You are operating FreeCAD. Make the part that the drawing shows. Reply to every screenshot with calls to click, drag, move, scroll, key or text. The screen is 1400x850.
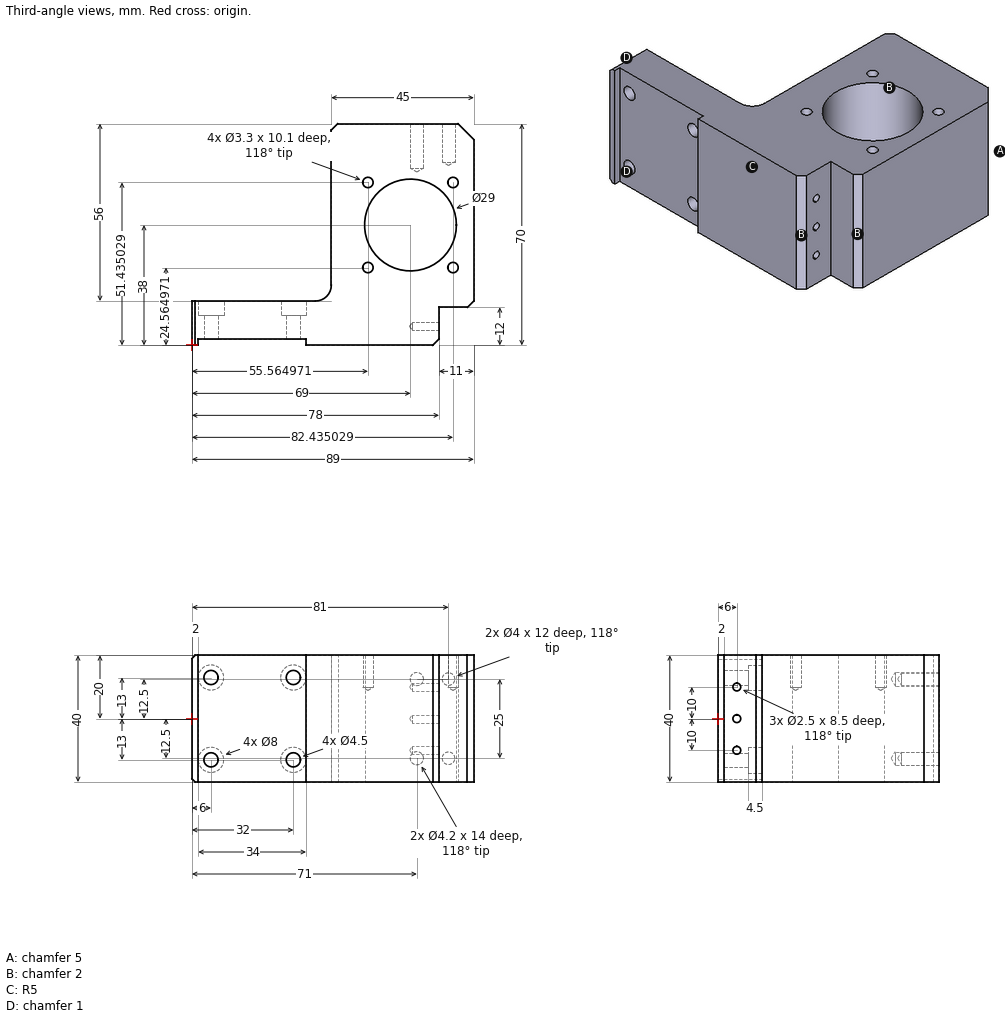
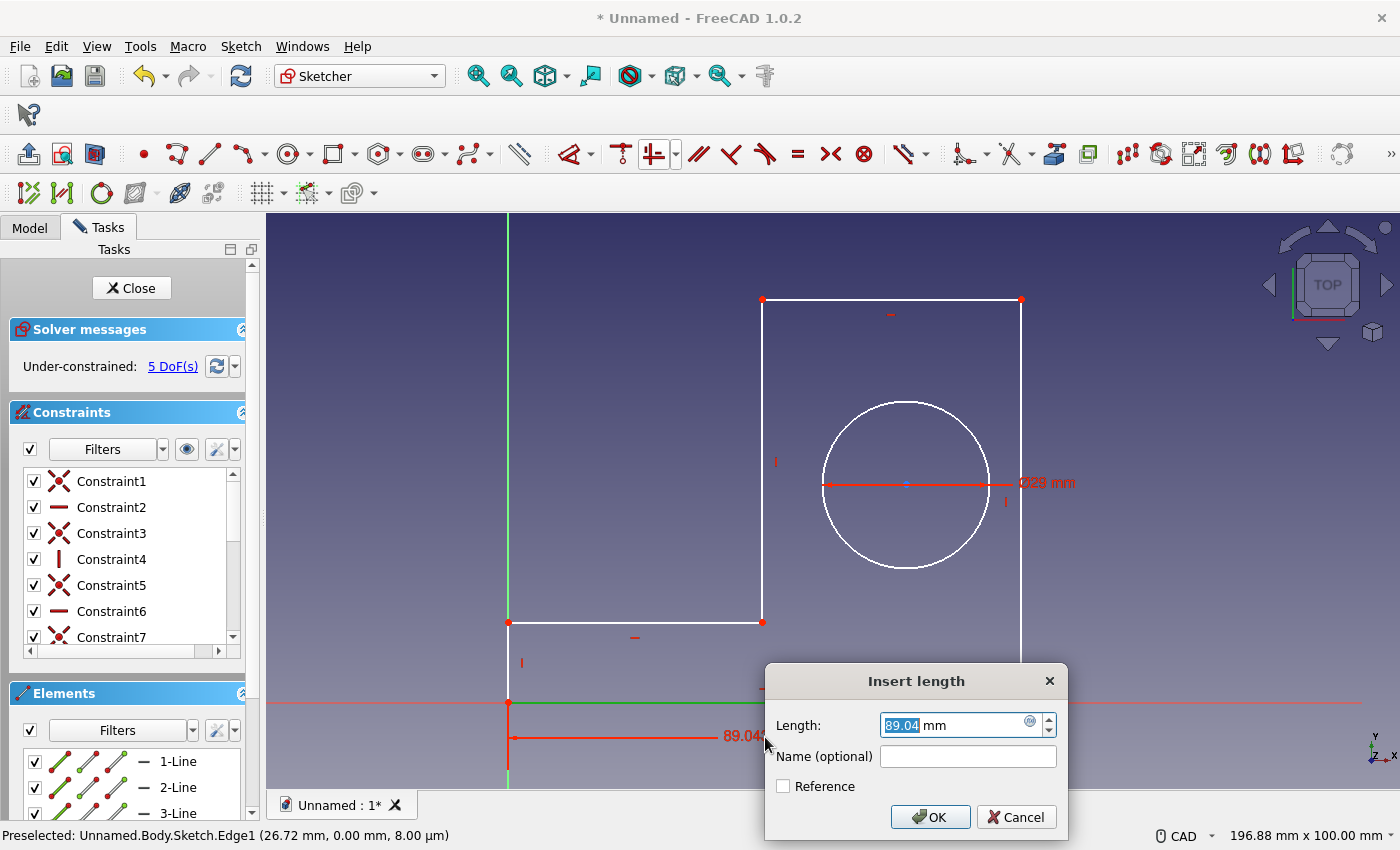
text(89)
key(Return)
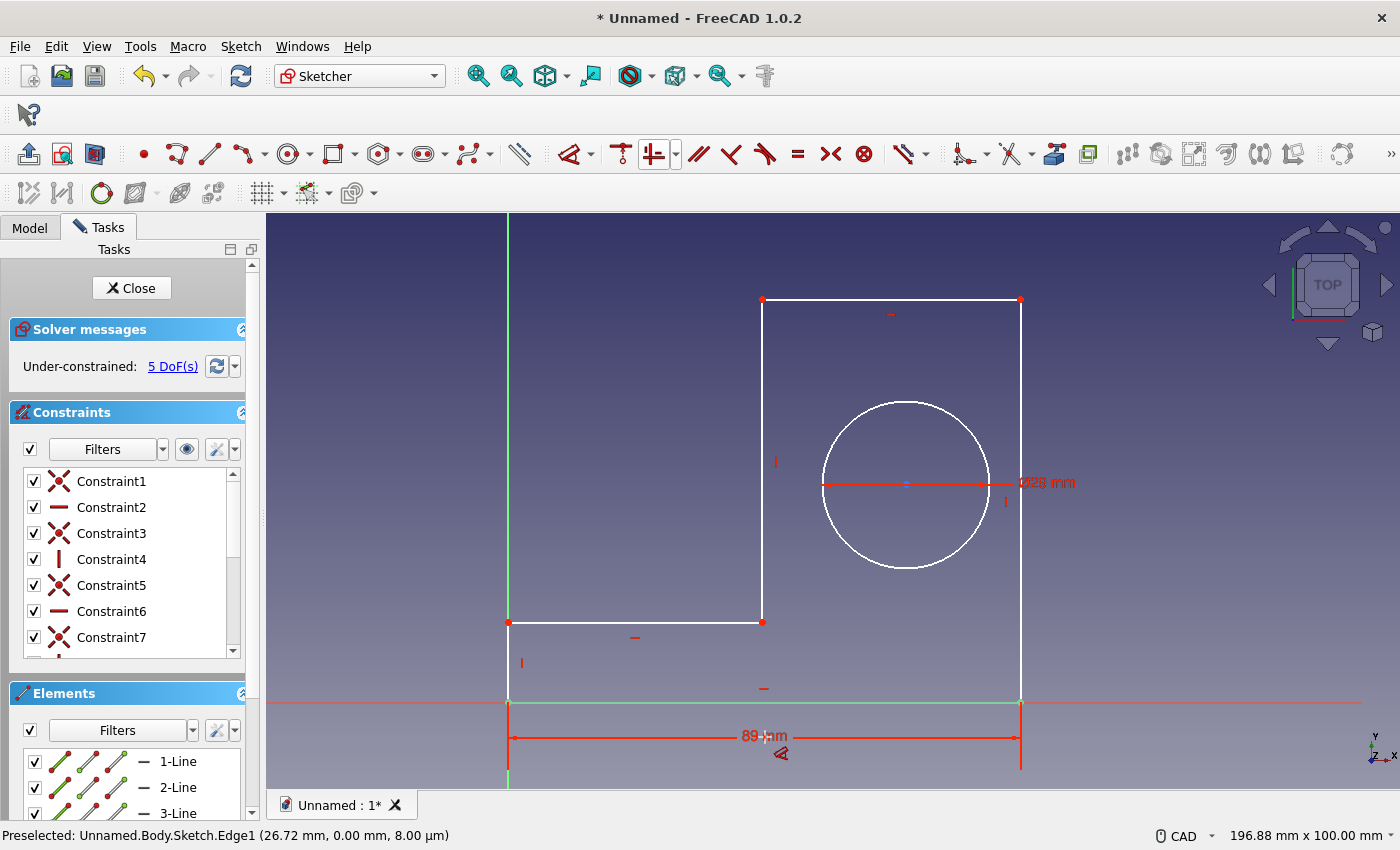
click(1021, 582)
click(1055, 501)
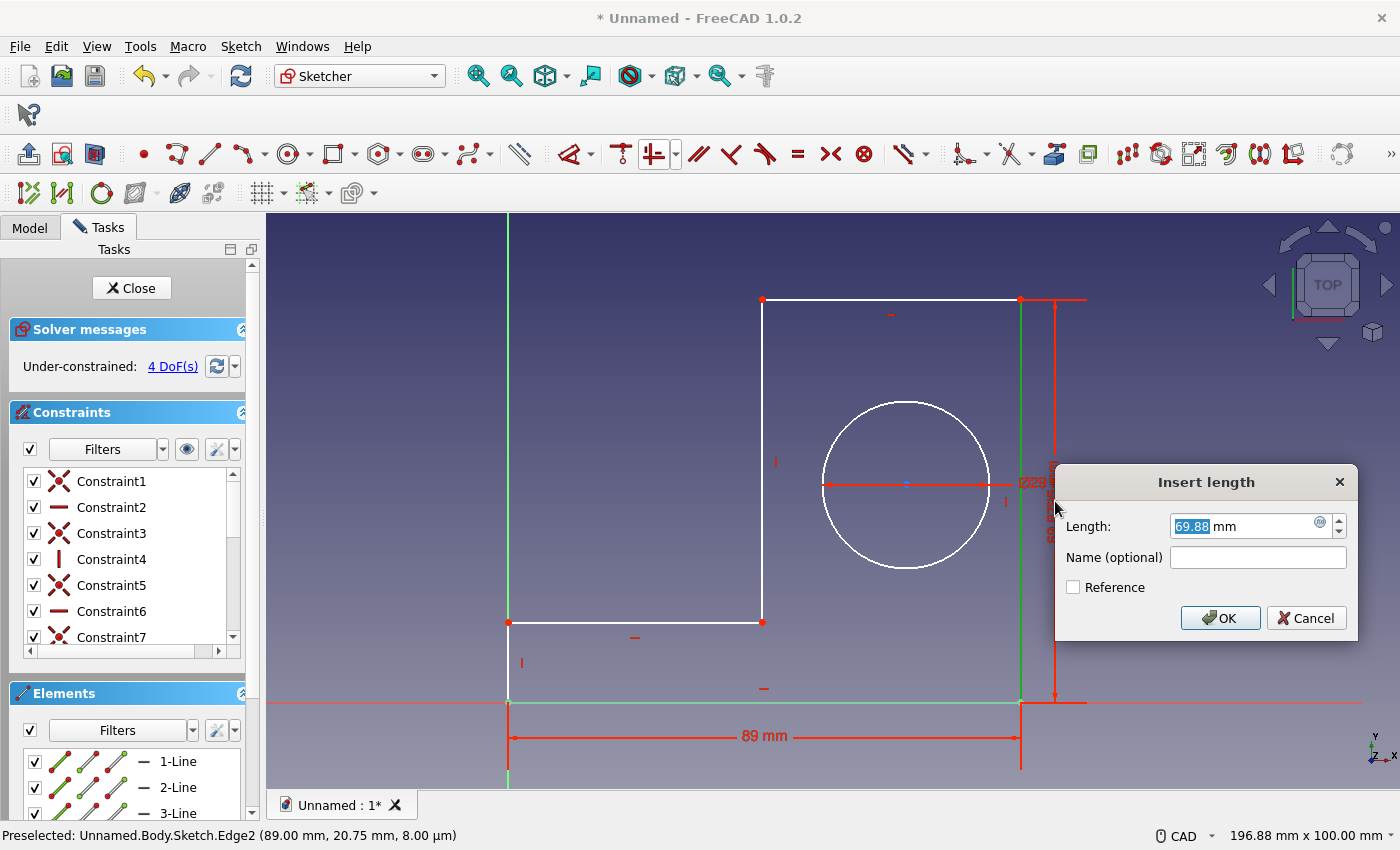
text(70)
key(Return)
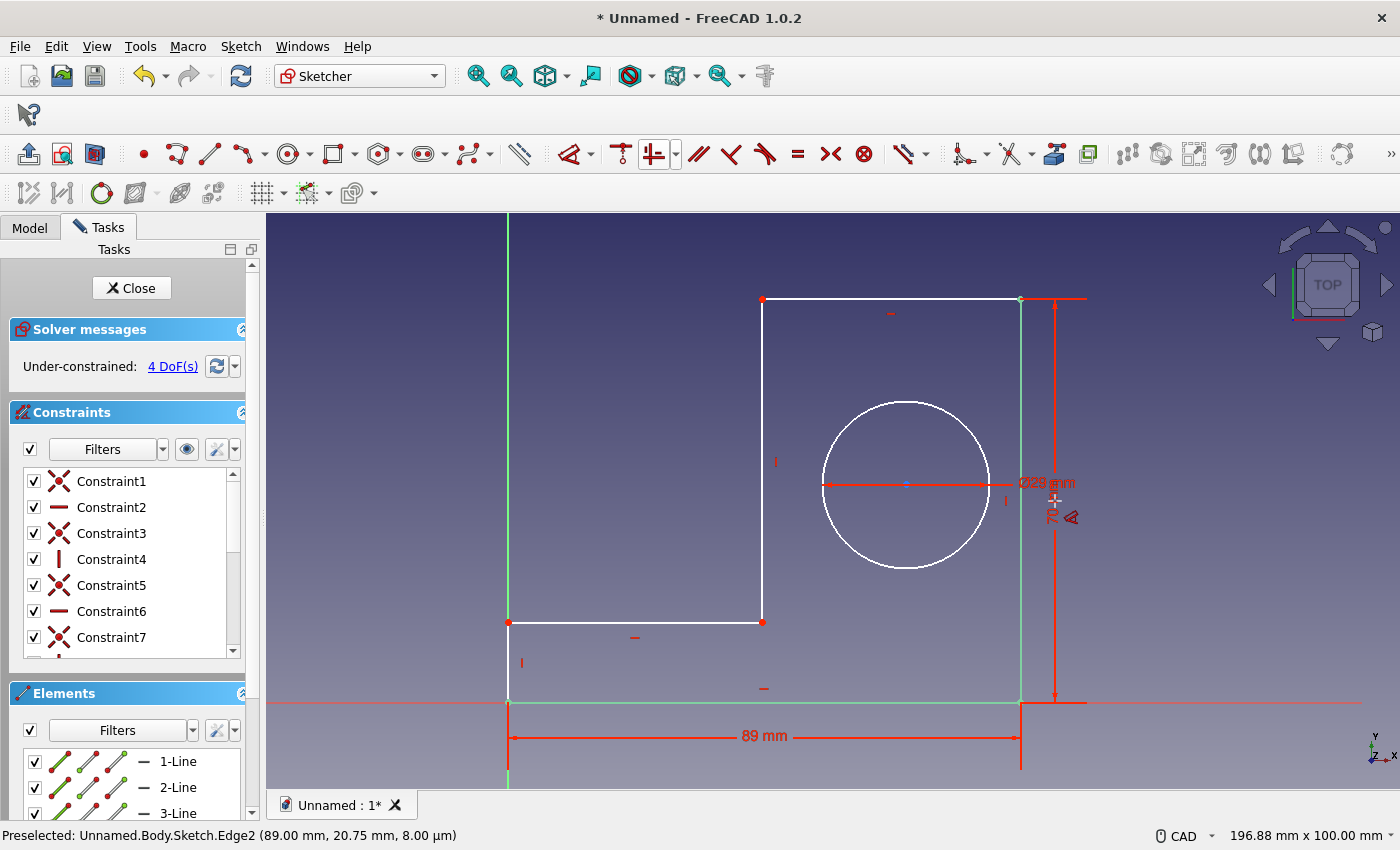
click(943, 299)
click(891, 265)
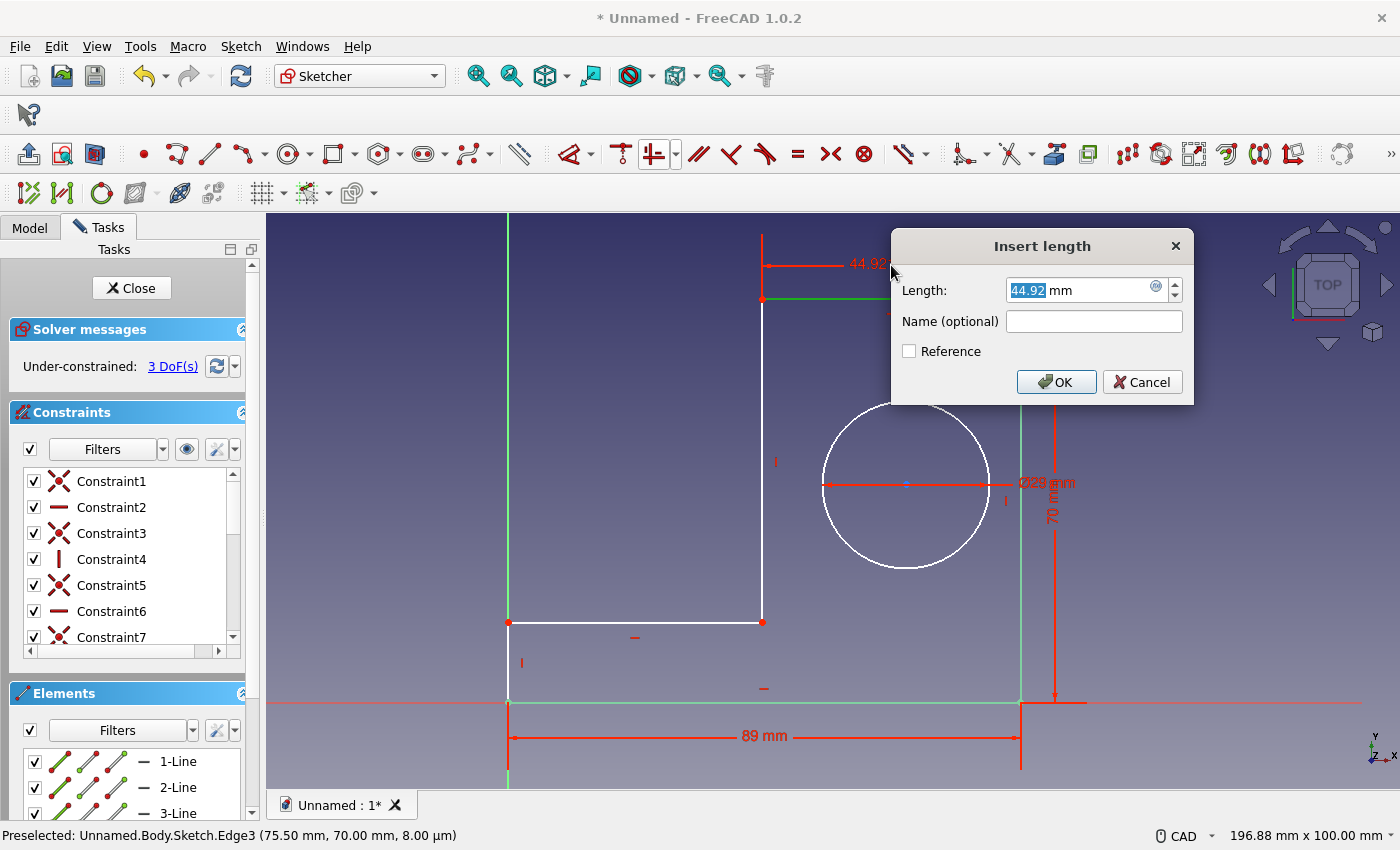
text(45)
key(Return)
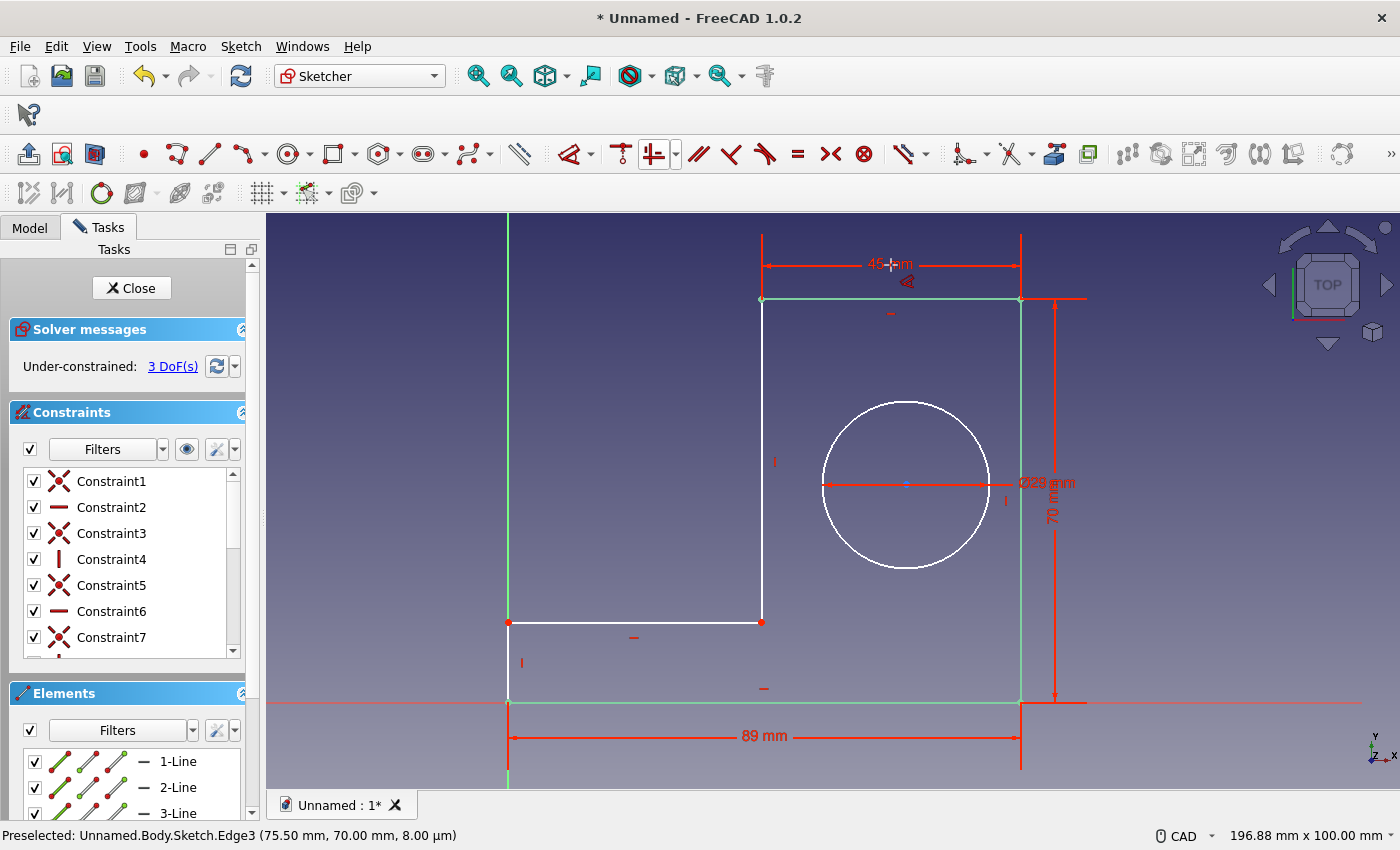
click(762, 396)
click(728, 461)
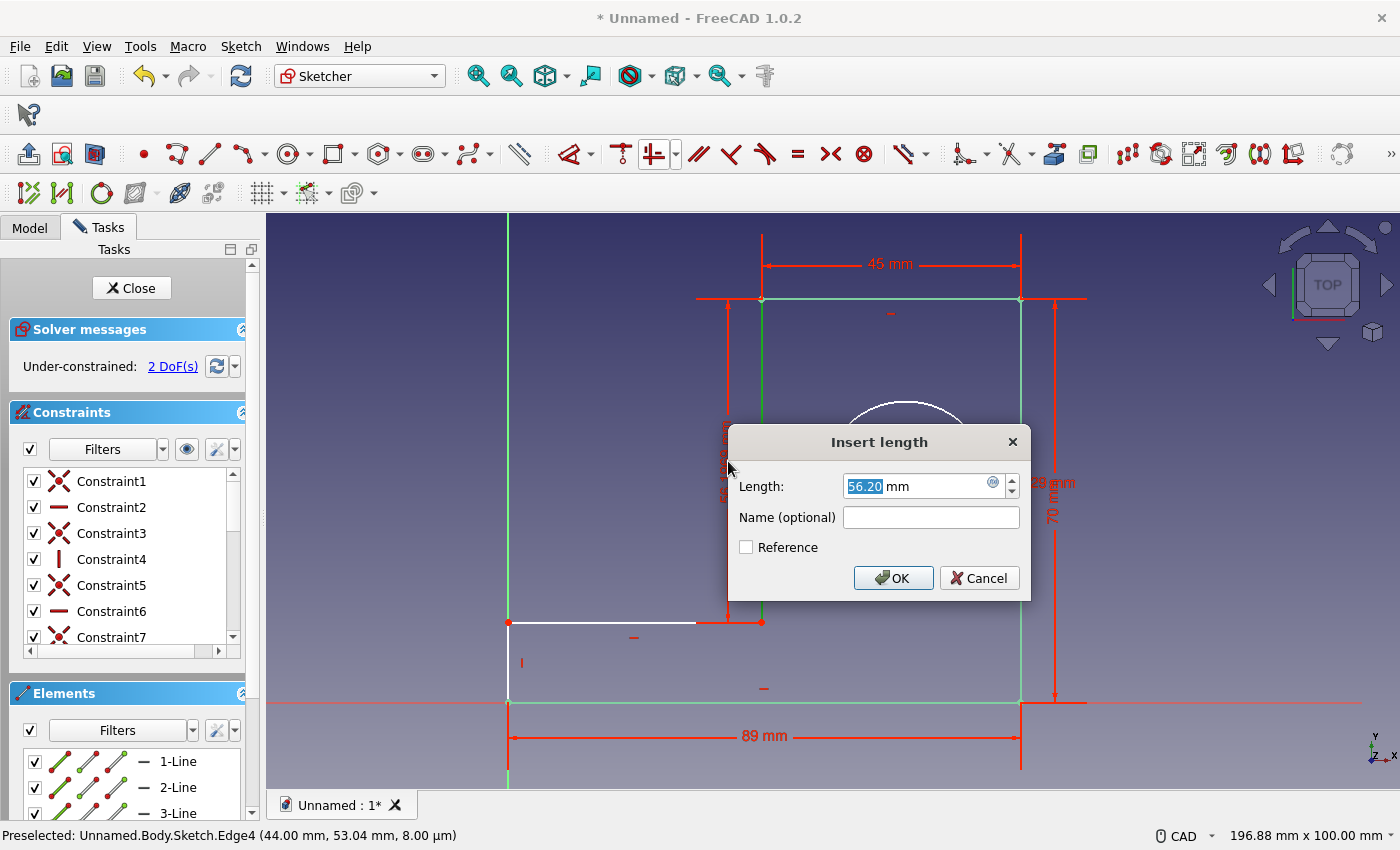
text(56)
key(Return)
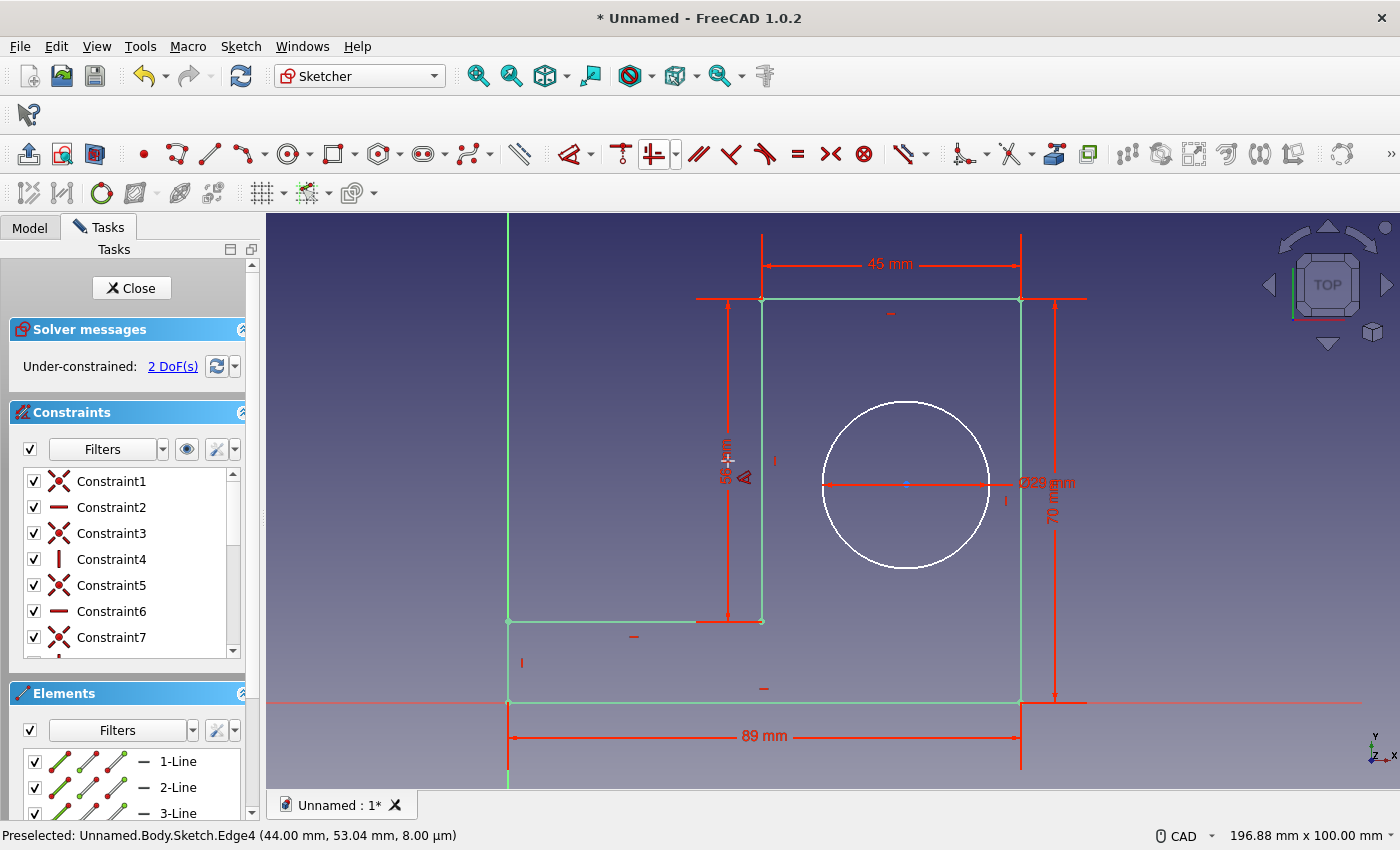
click(906, 485)
click(616, 737)